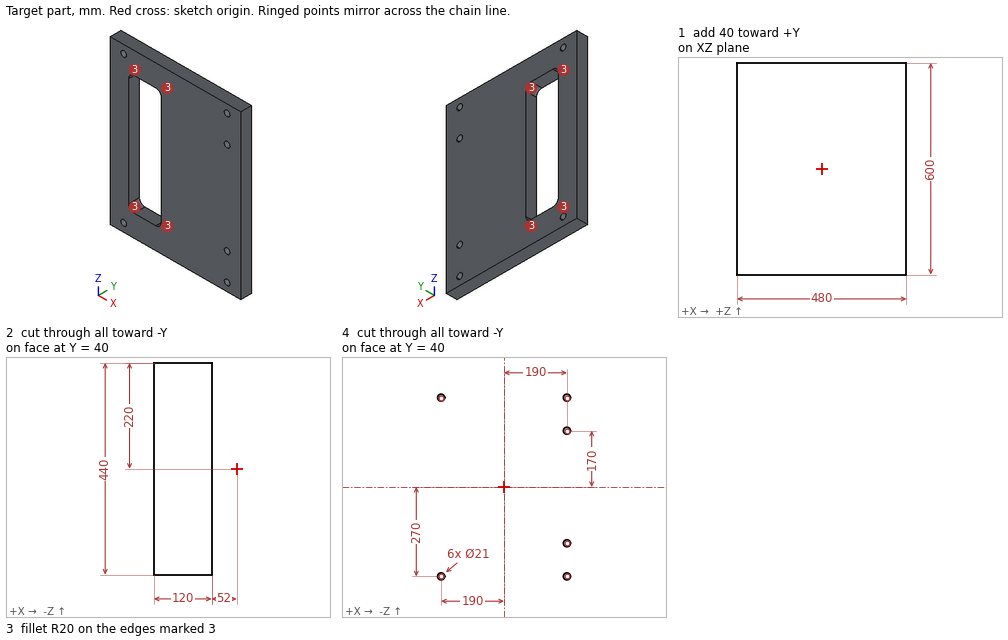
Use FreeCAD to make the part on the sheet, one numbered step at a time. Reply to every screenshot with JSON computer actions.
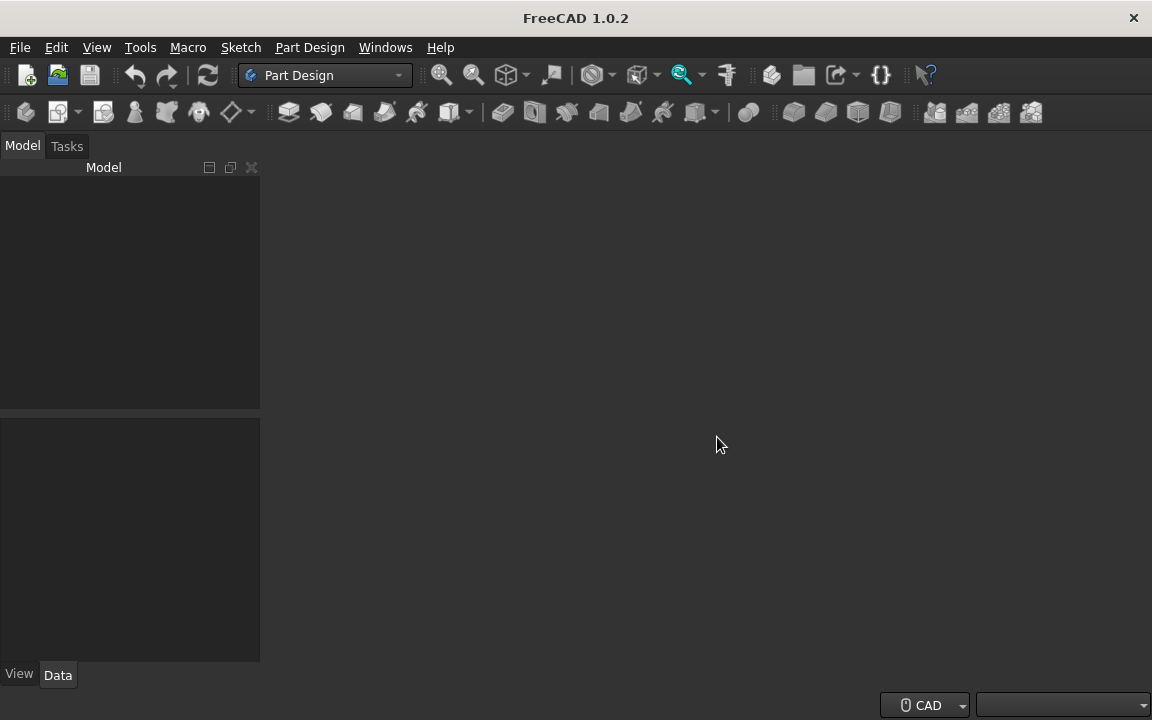
{"action": "left_click", "coordinate": [26, 76]}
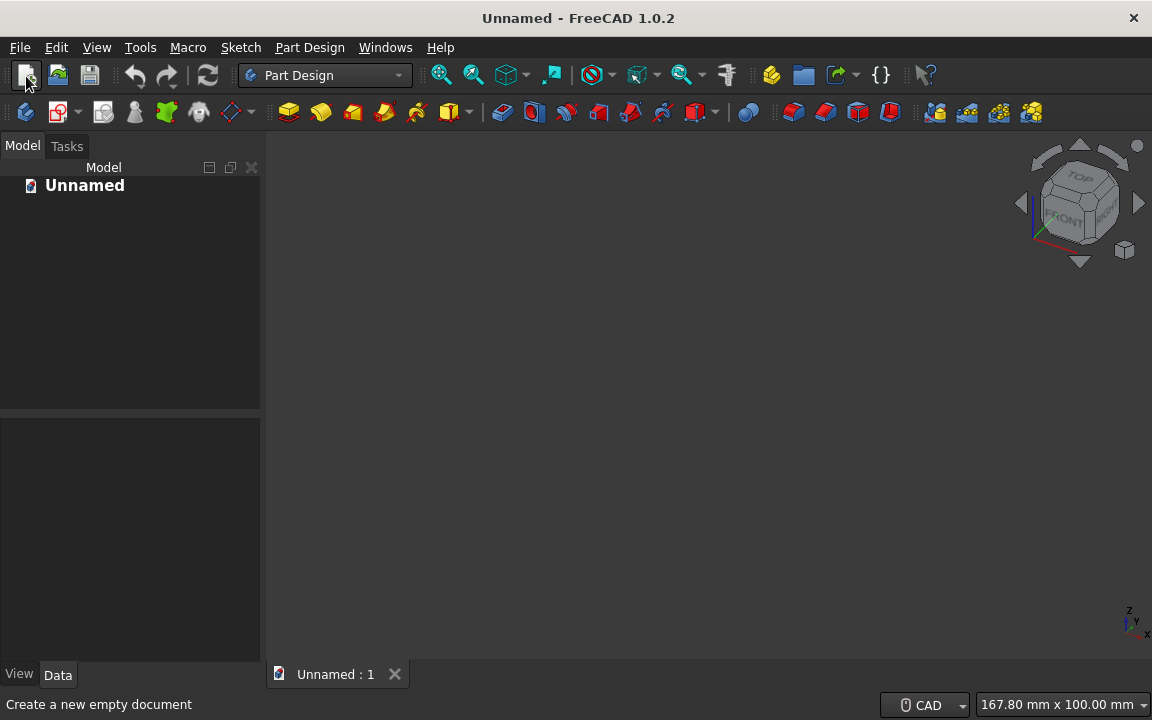
{"action": "left_click", "coordinate": [58, 112]}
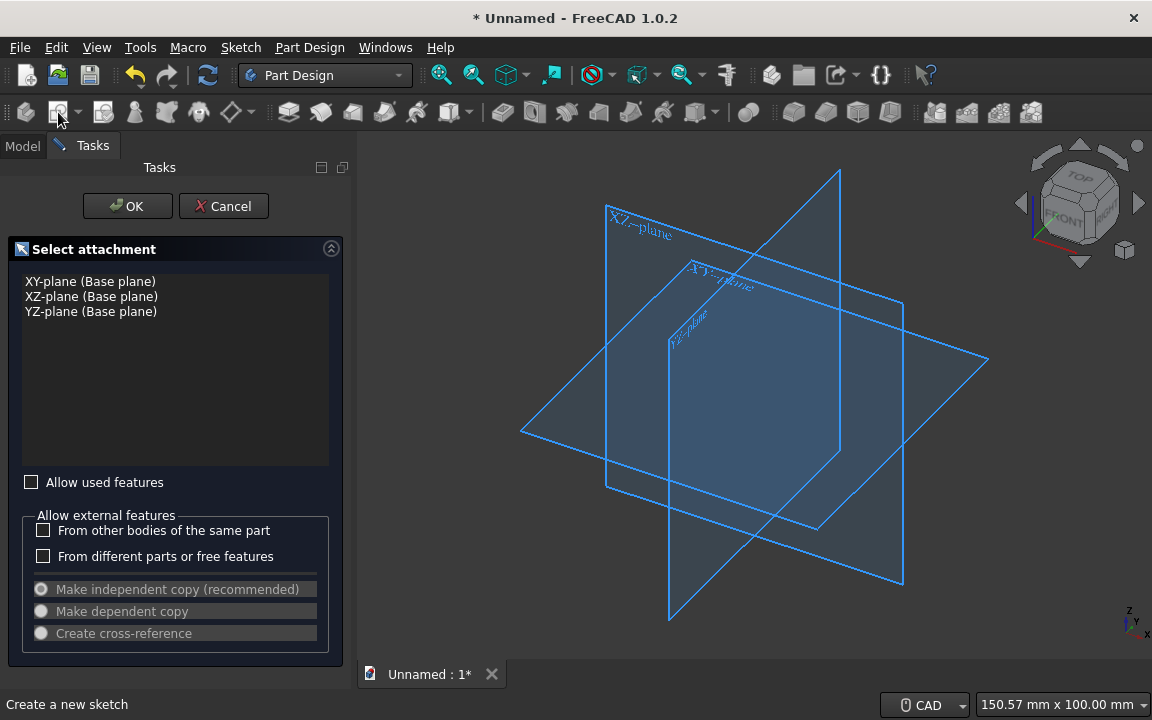
{"action": "left_click", "coordinate": [82, 296]}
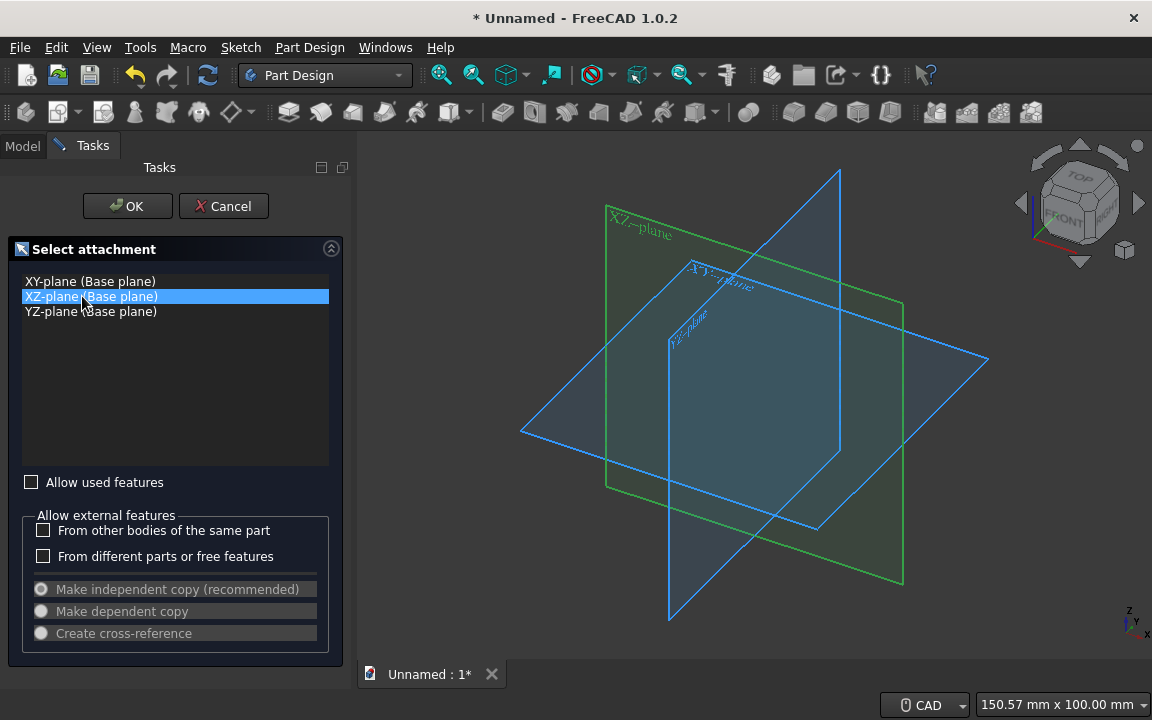
{"action": "left_click", "coordinate": [128, 206]}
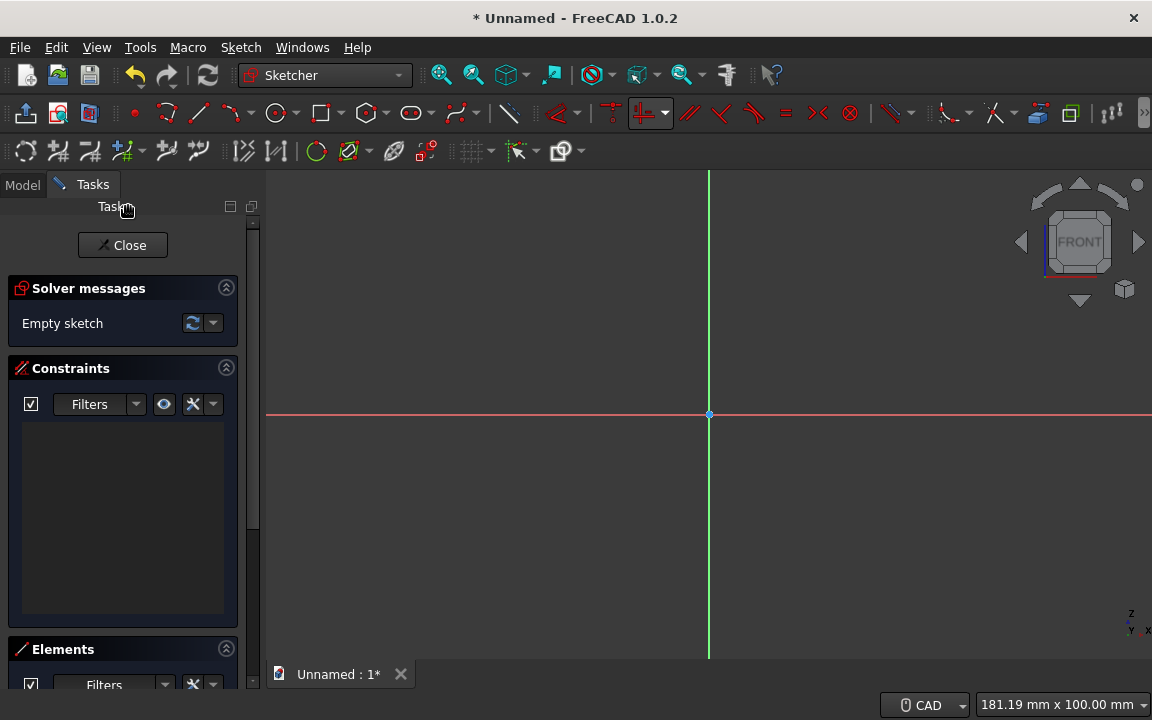
{"action": "scroll", "coordinate": [632, 414], "scroll_direction": "down", "scroll_amount": 11}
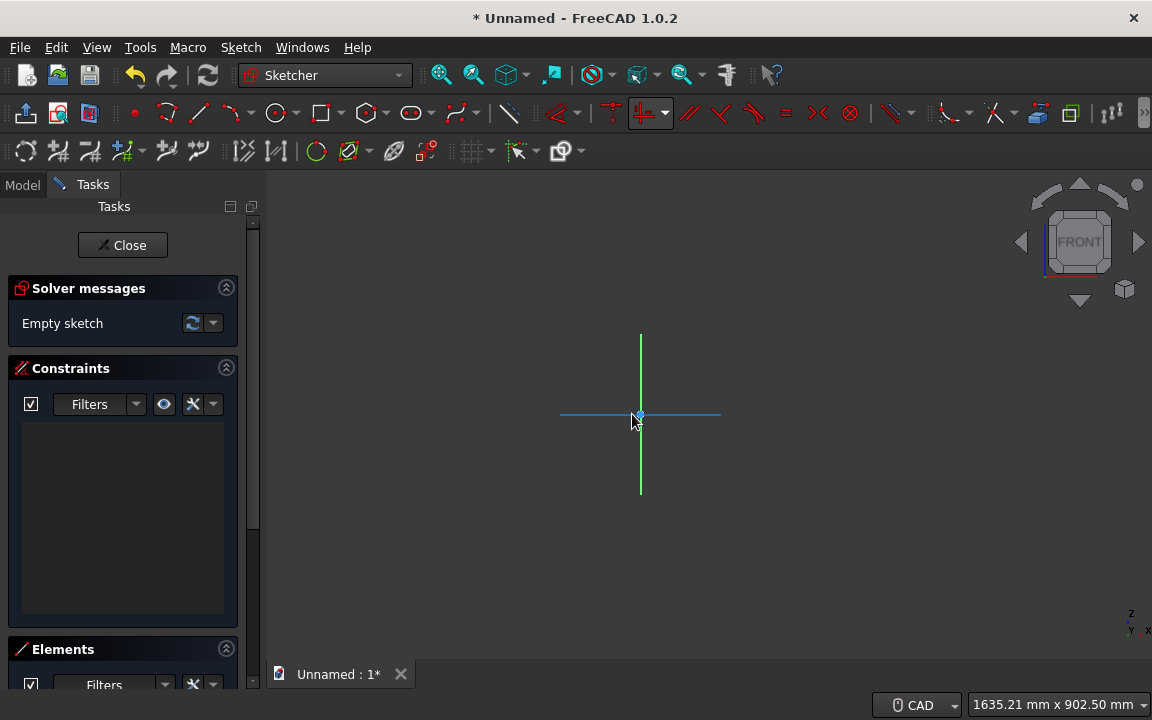
{"action": "key", "text": "g v"}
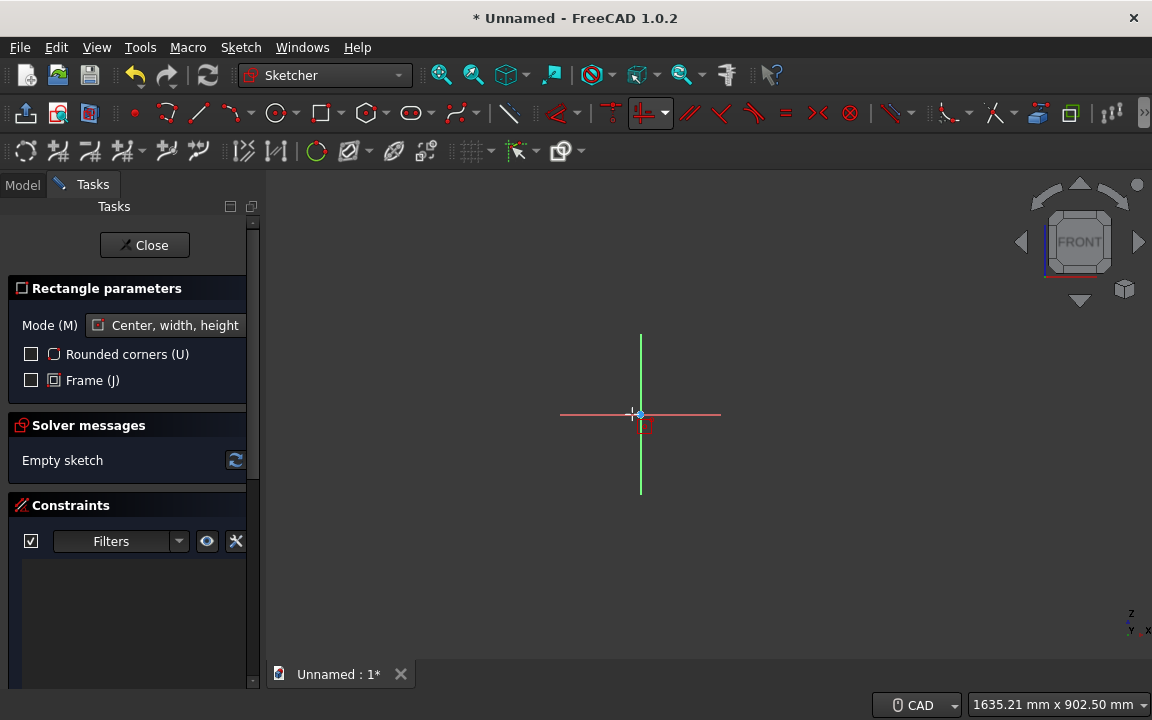
{"action": "left_click", "coordinate": [641, 414]}
{"action": "left_click", "coordinate": [771, 252]}
{"action": "key", "text": "Escape"}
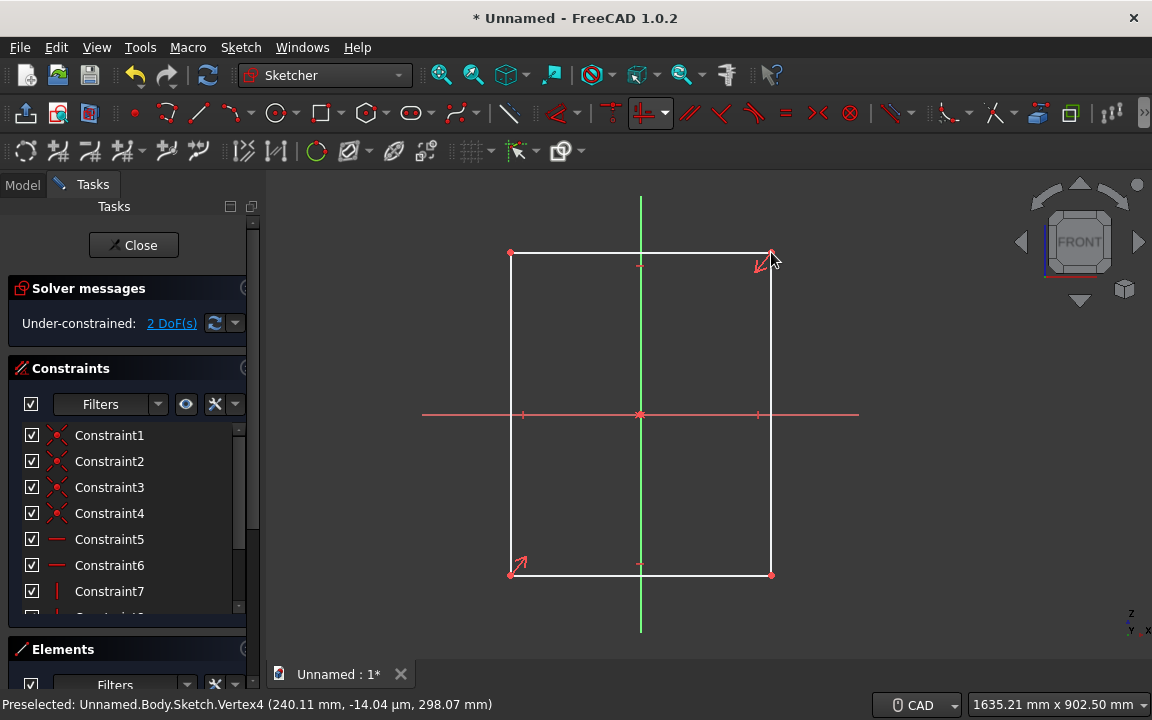
{"action": "left_click", "coordinate": [589, 576]}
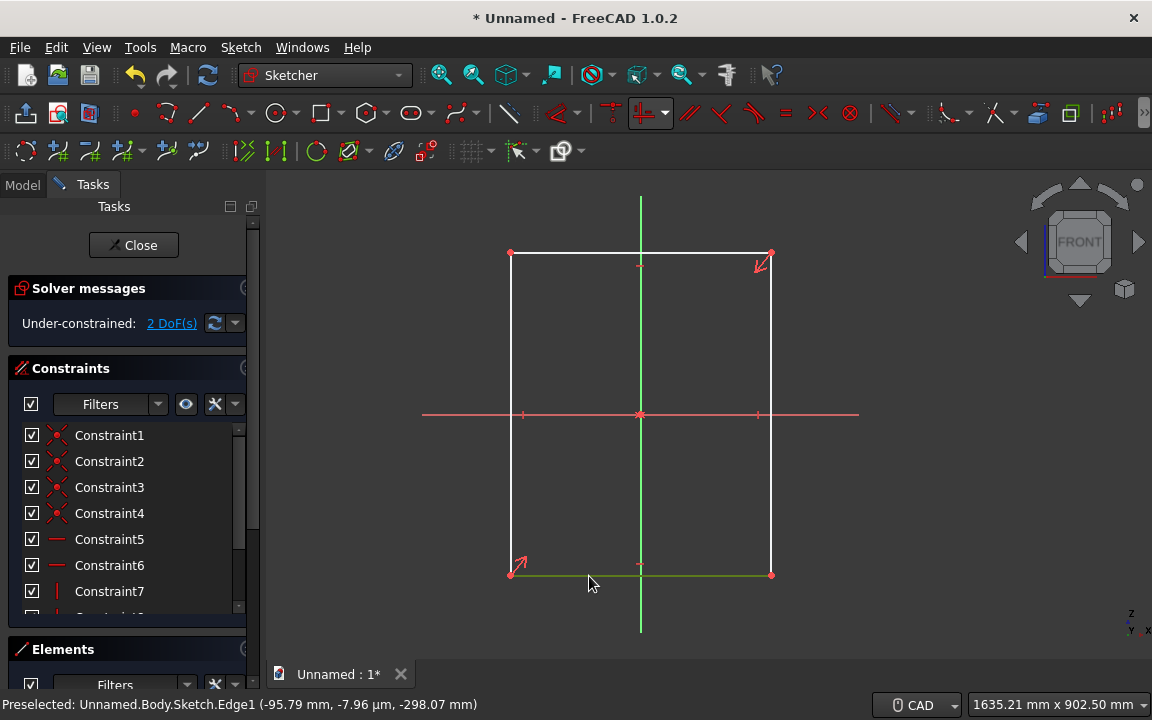
{"action": "key", "text": "l"}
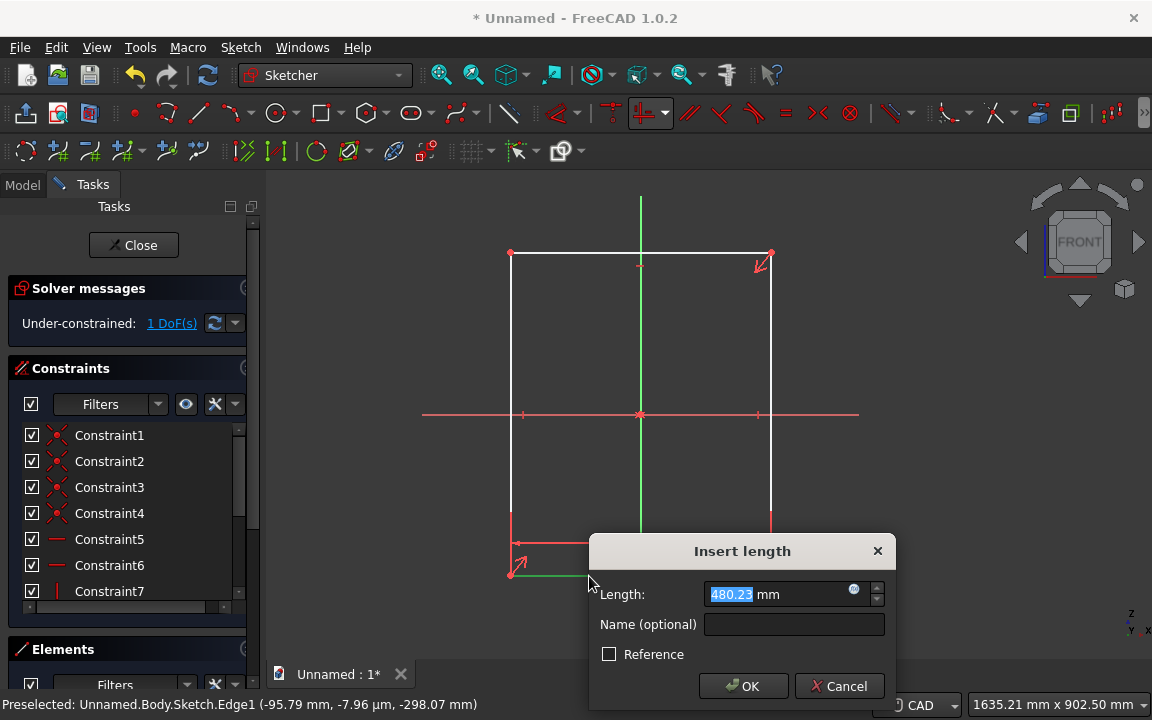
{"action": "type", "text": "480"}
{"action": "key", "text": "Return"}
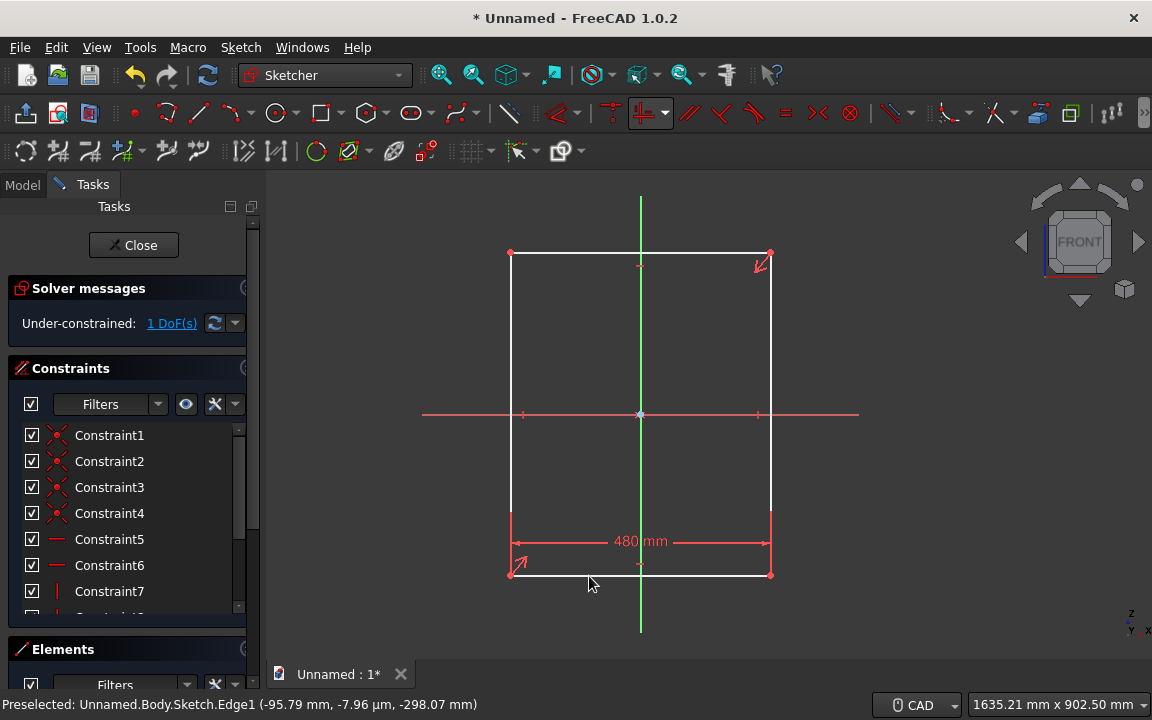
{"action": "left_click", "coordinate": [771, 479]}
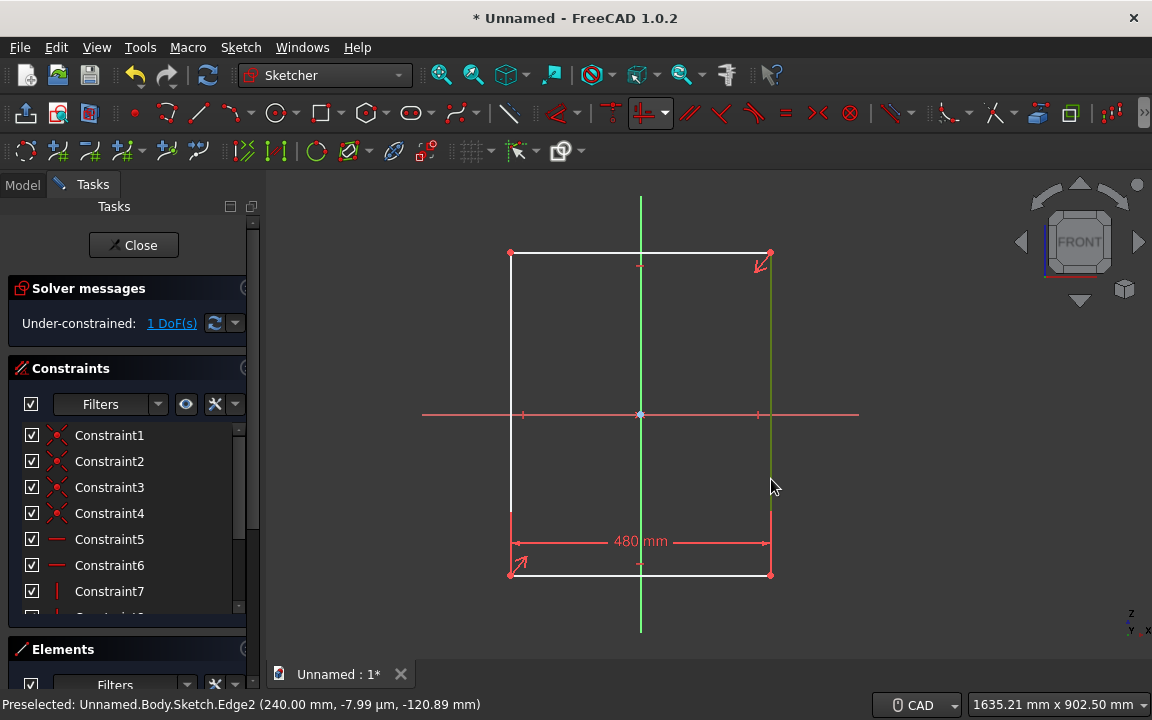
{"action": "key", "text": "i"}